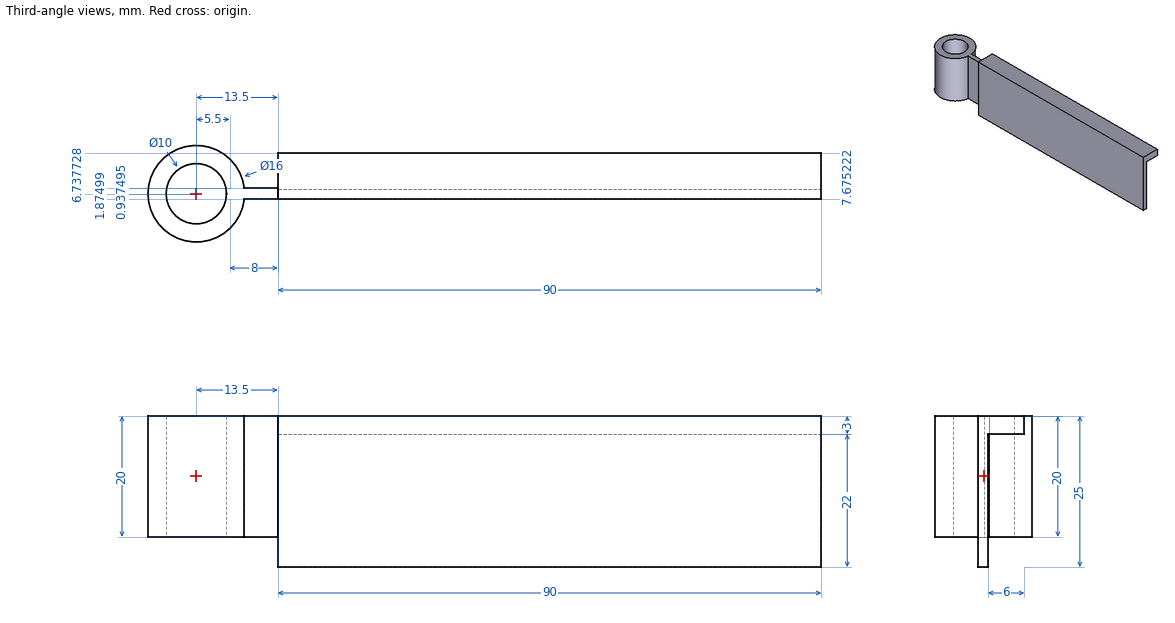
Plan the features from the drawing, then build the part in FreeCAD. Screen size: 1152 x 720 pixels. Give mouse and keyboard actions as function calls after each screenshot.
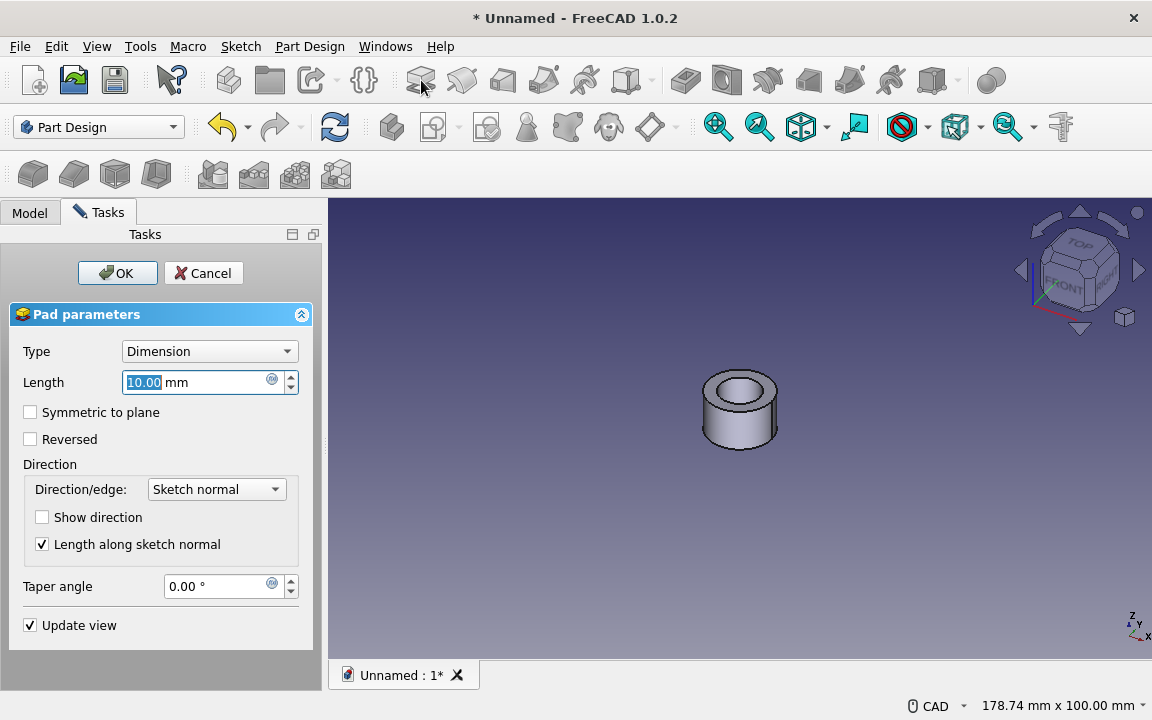
text(20)
key(Tab)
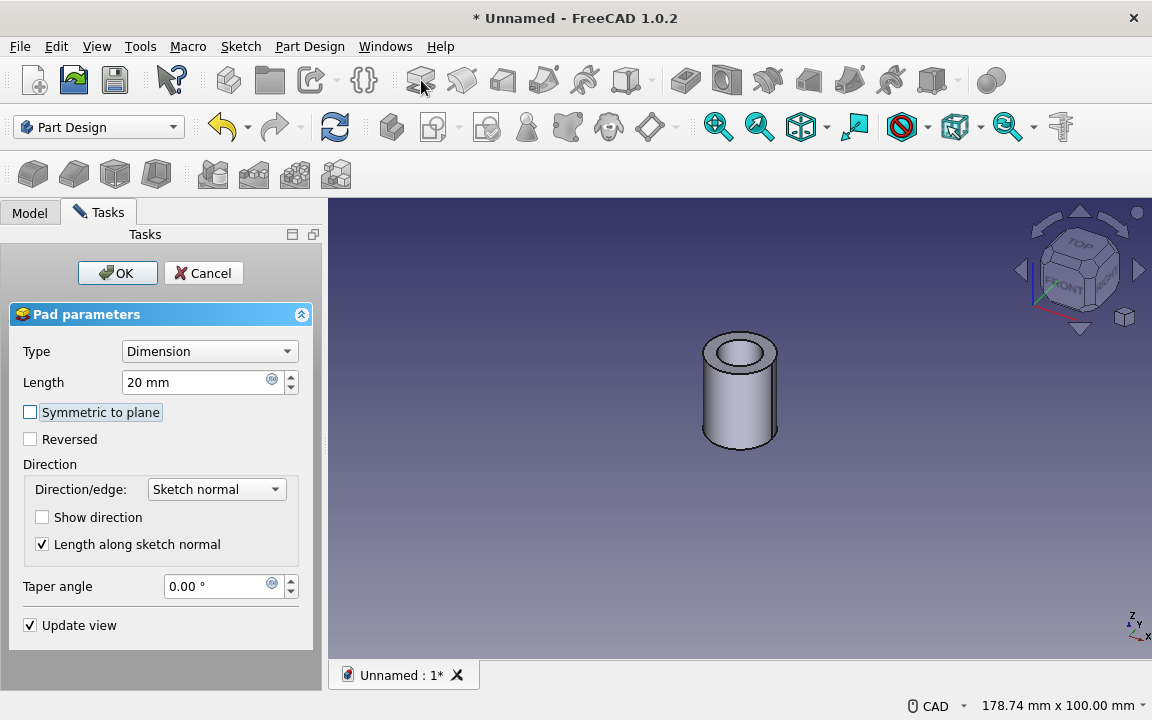
click(31, 412)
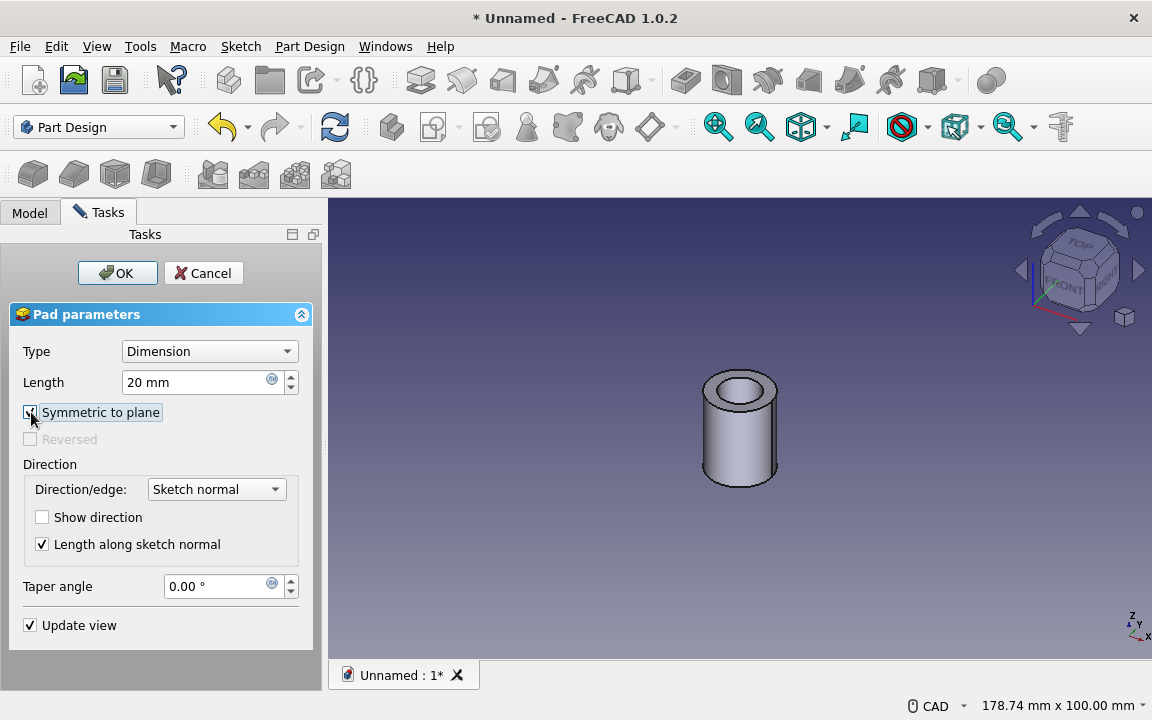
click(118, 273)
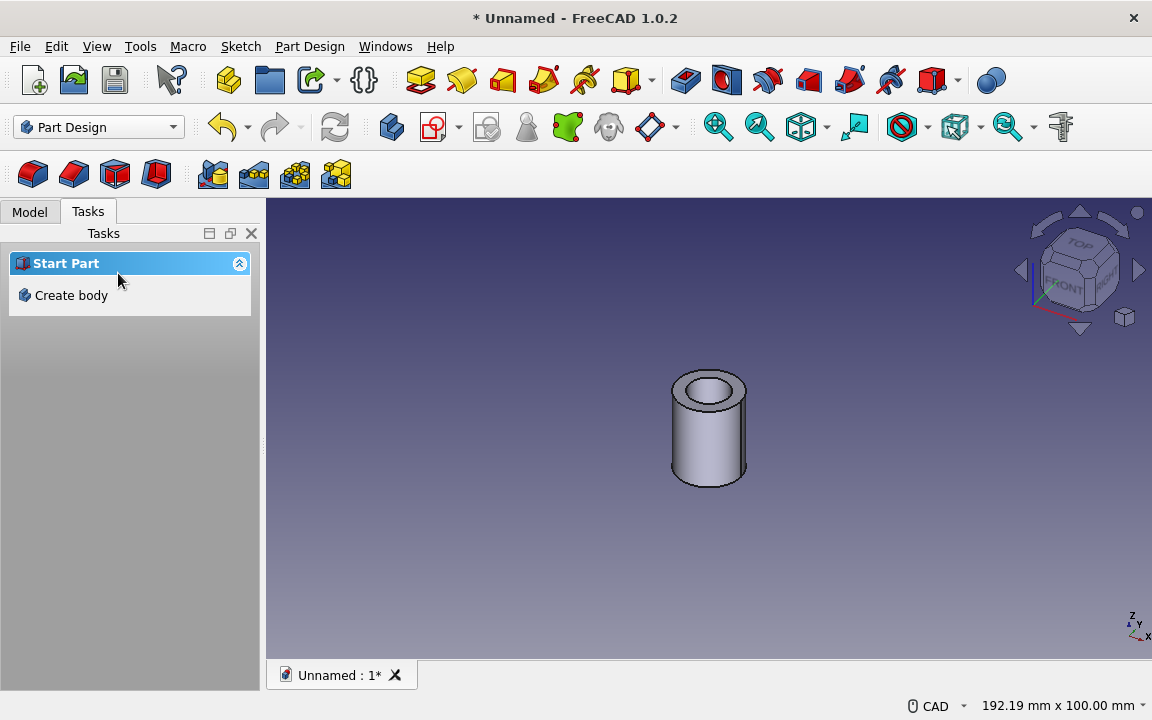
click(719, 128)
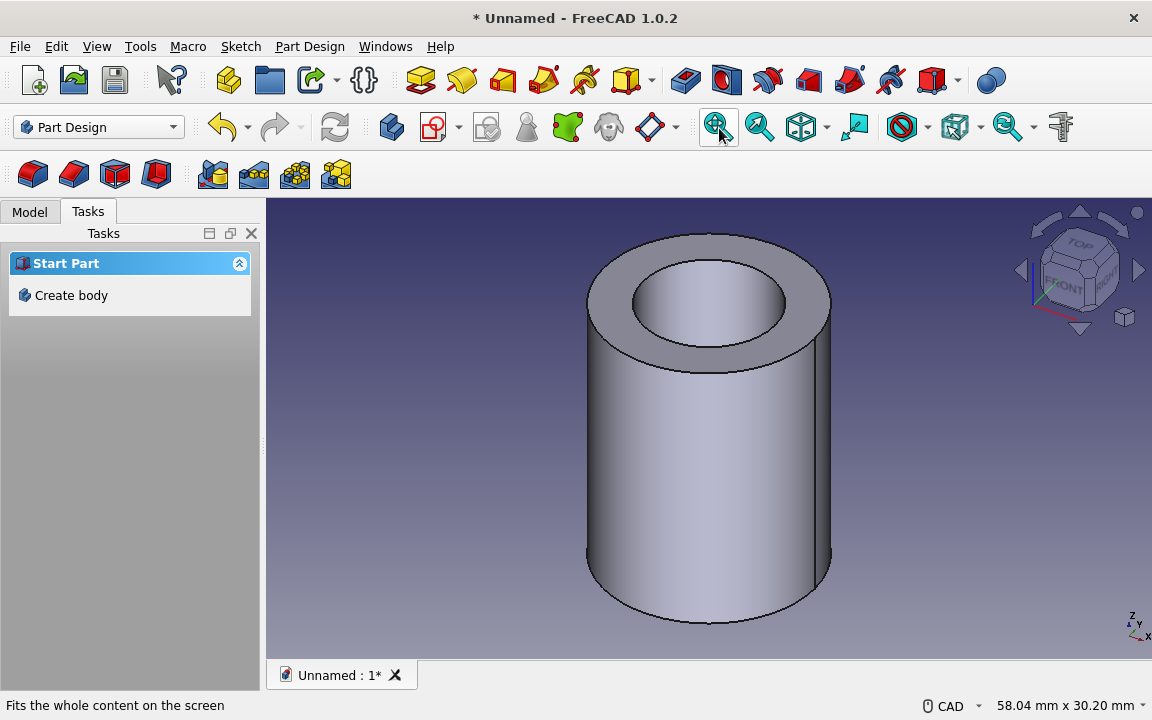
click(432, 128)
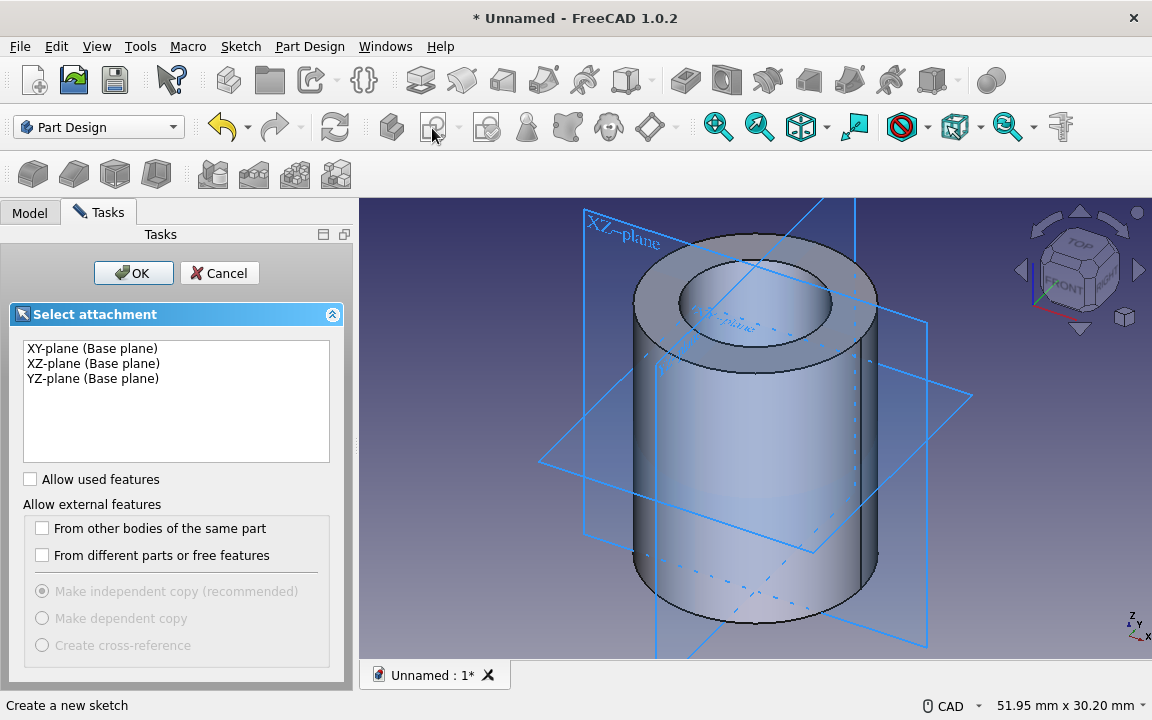
click(84, 348)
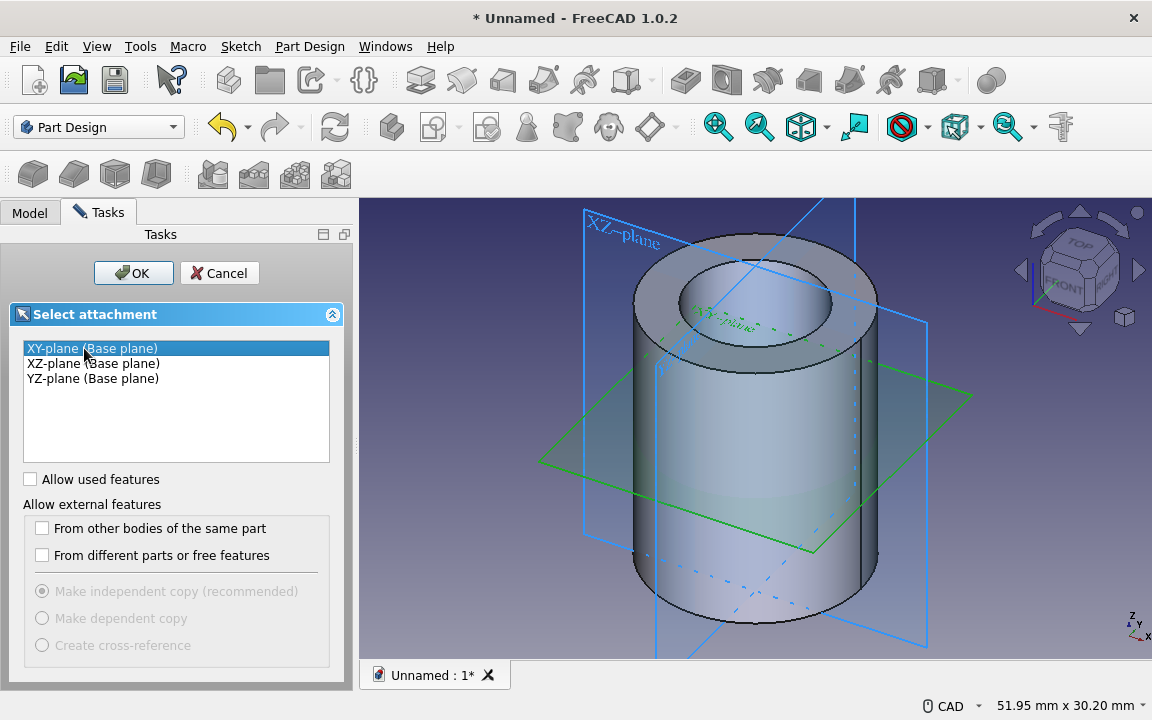
click(134, 273)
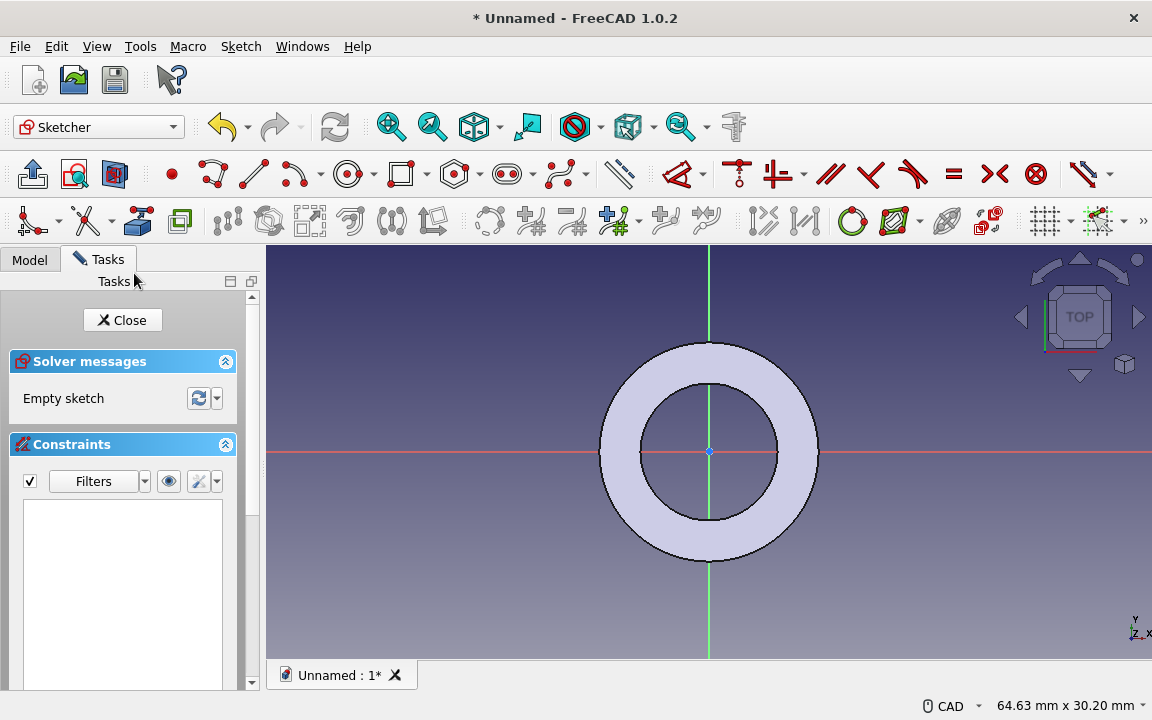
click(115, 174)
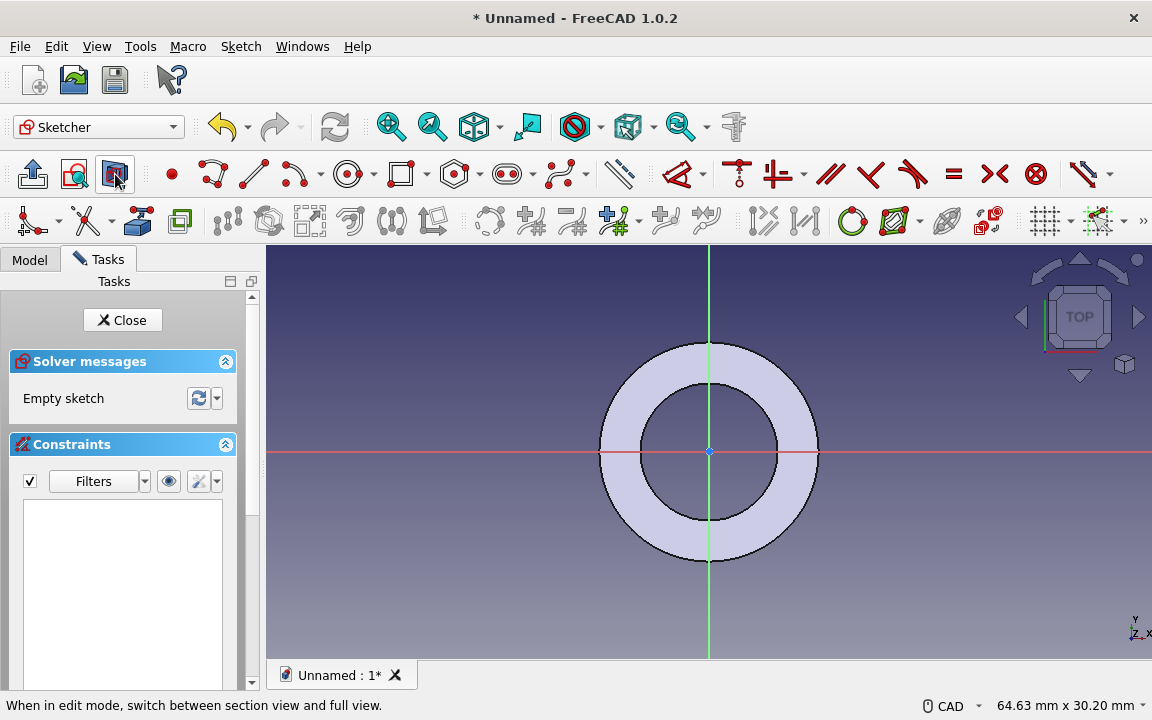
scroll(895, 452, up, 5)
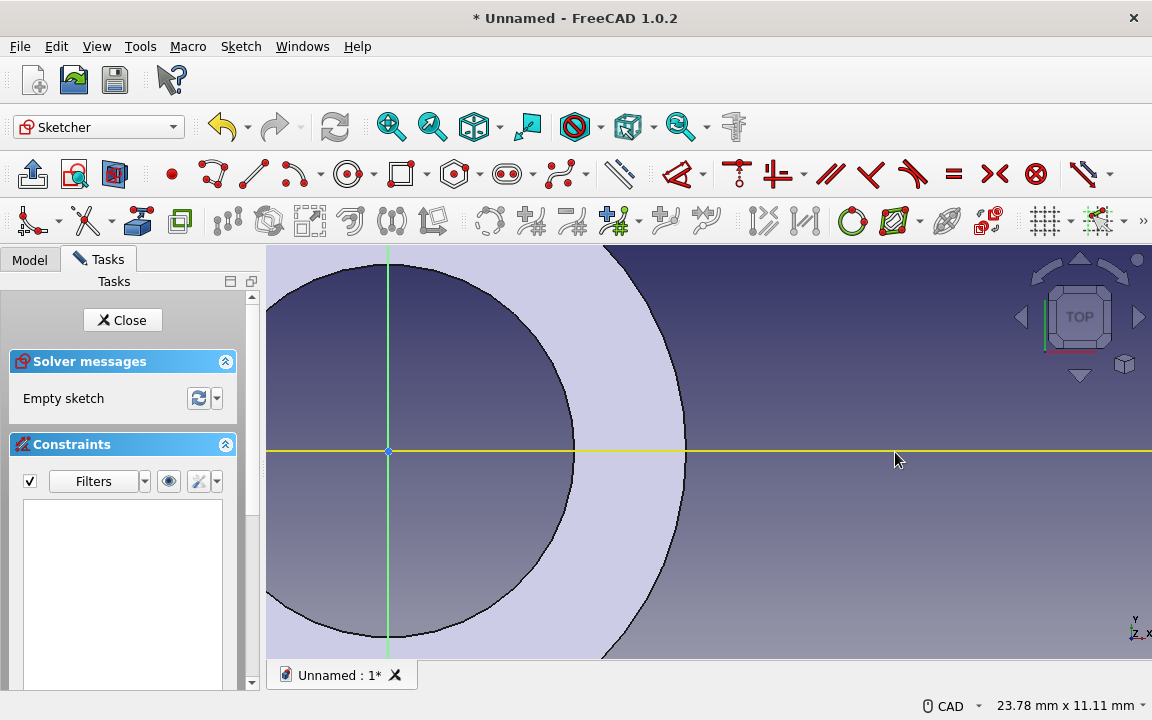
click(400, 174)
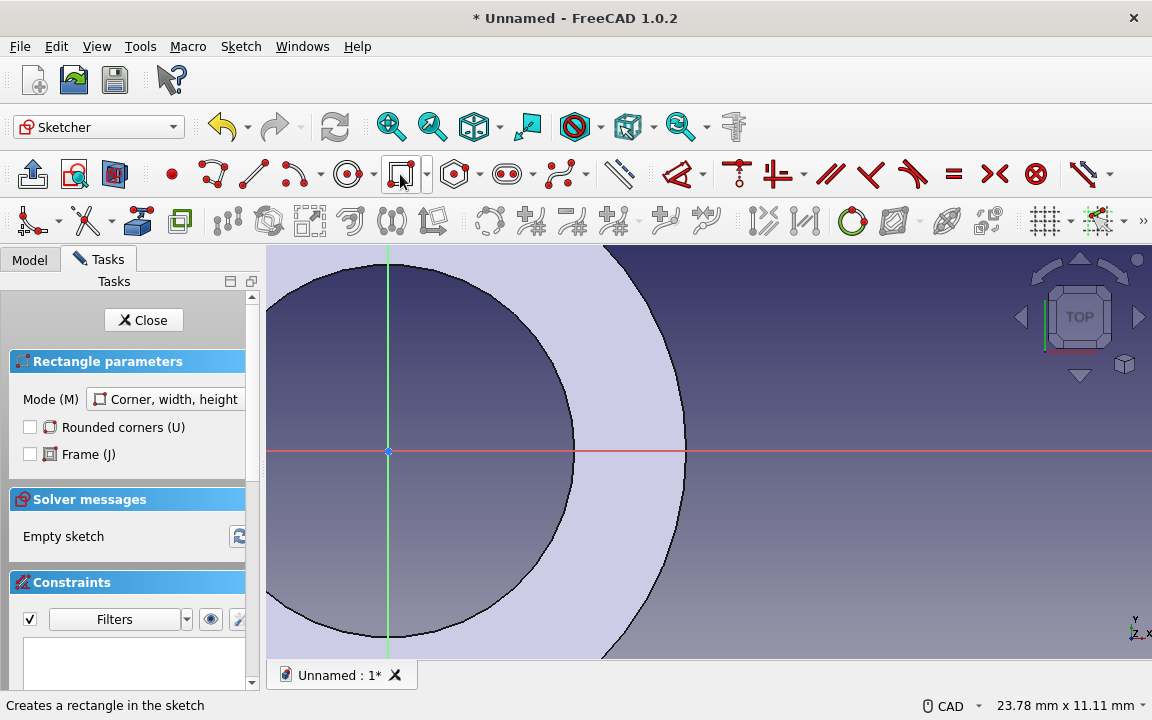
click(593, 416)
move(891, 486)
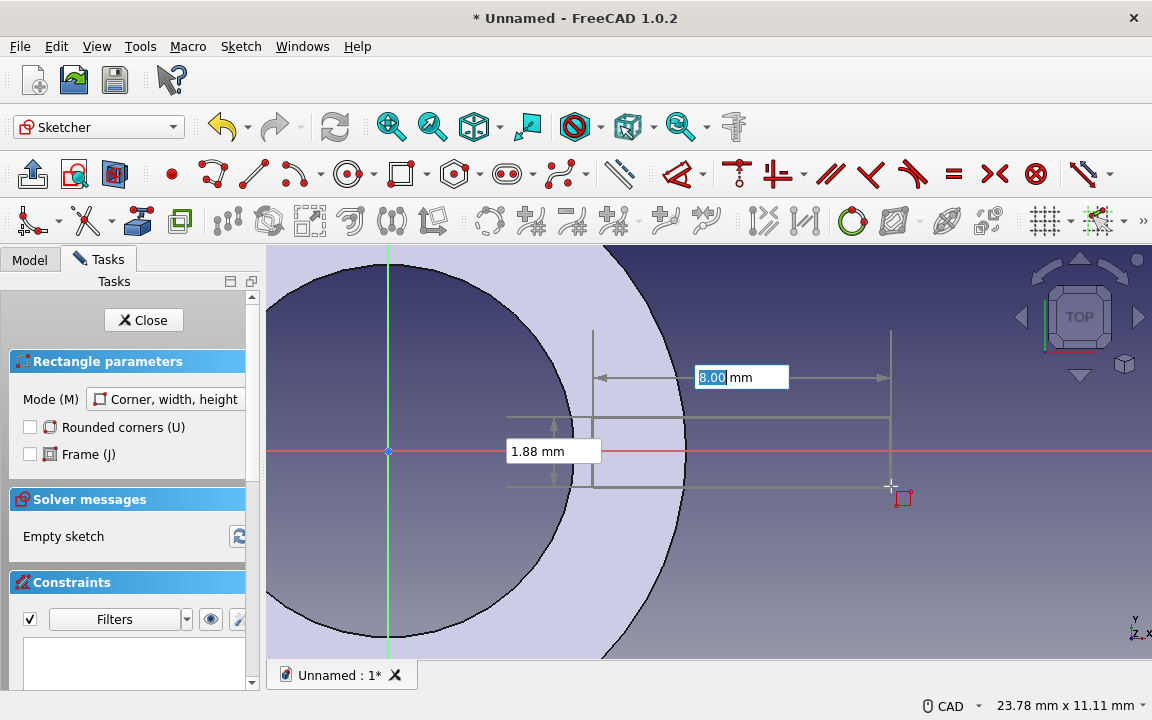
text(8)
key(Tab)
text(1.87499)
key(Return)
key(Escape)